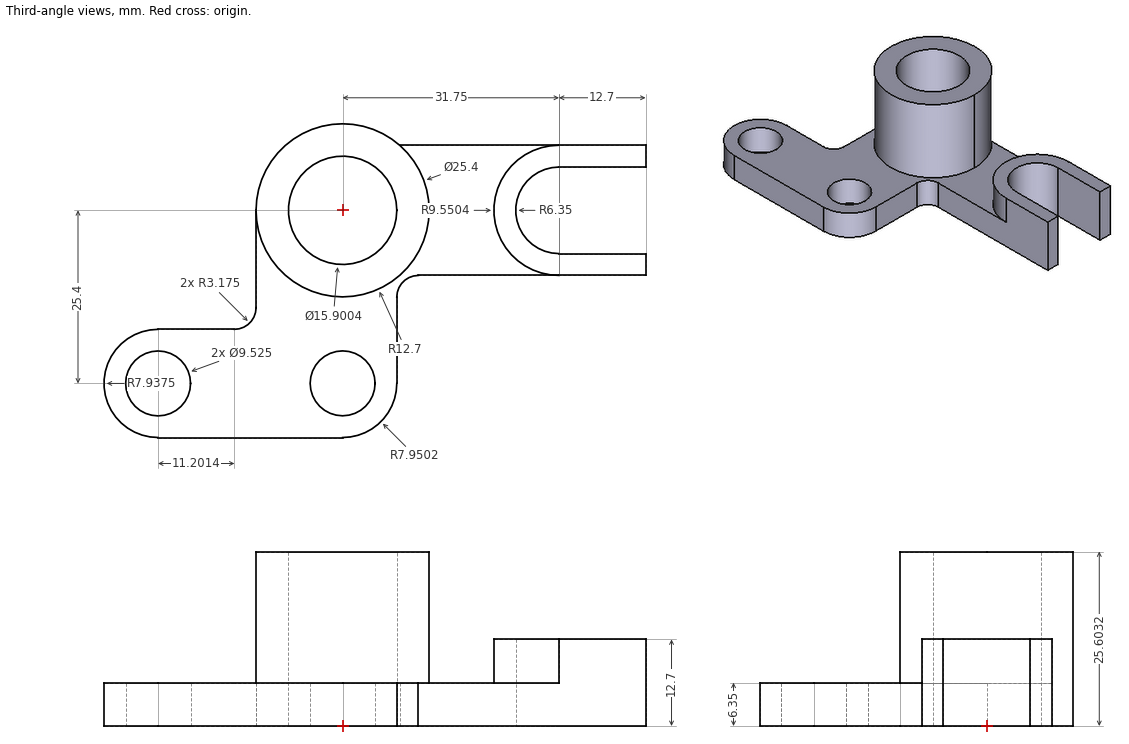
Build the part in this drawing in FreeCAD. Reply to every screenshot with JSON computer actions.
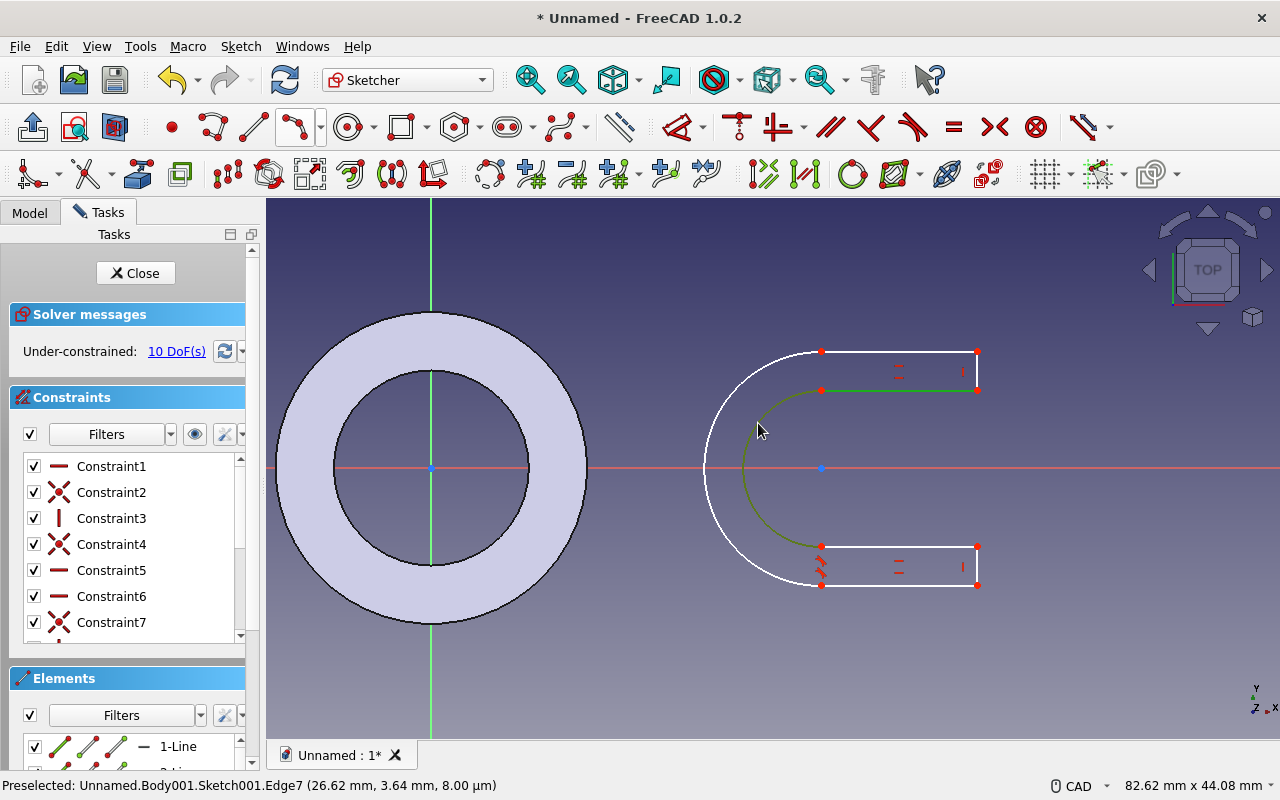
{"action": "left_click", "coordinate": [913, 128]}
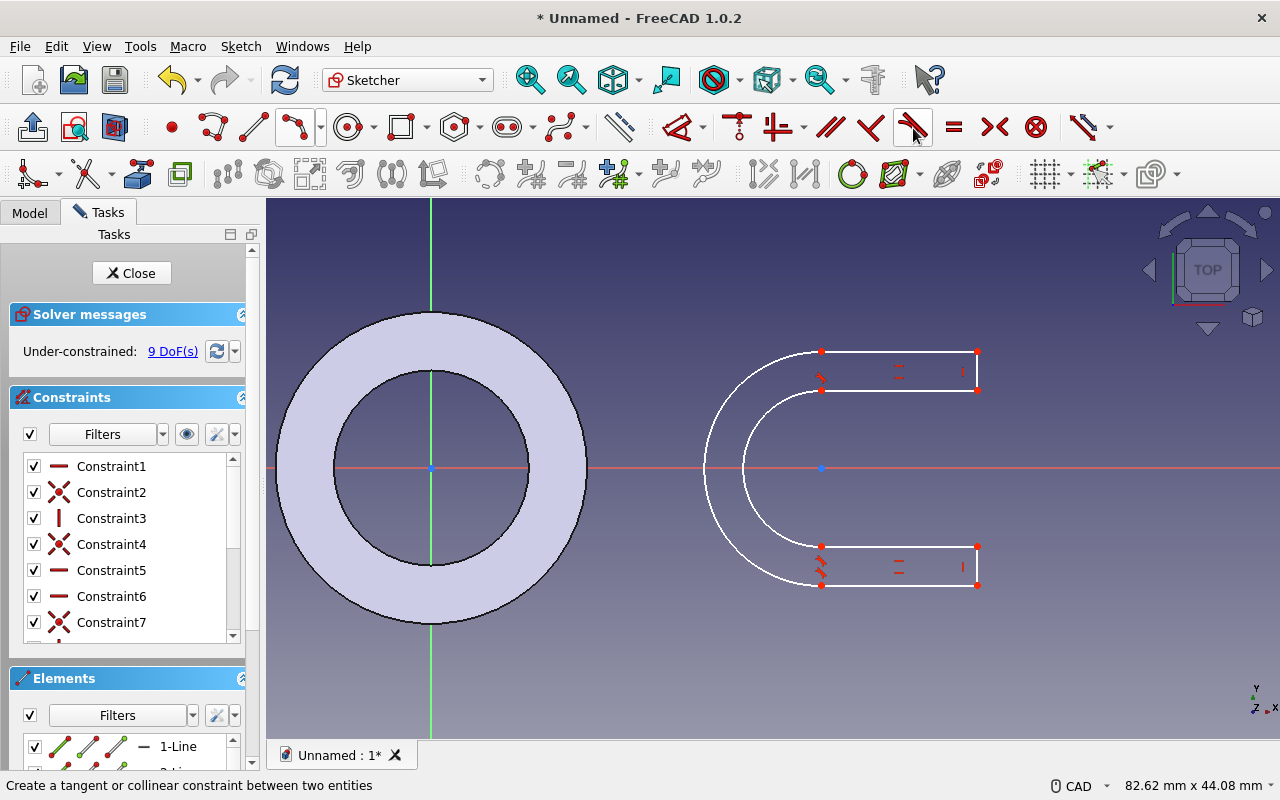
{"action": "left_click", "coordinate": [930, 352]}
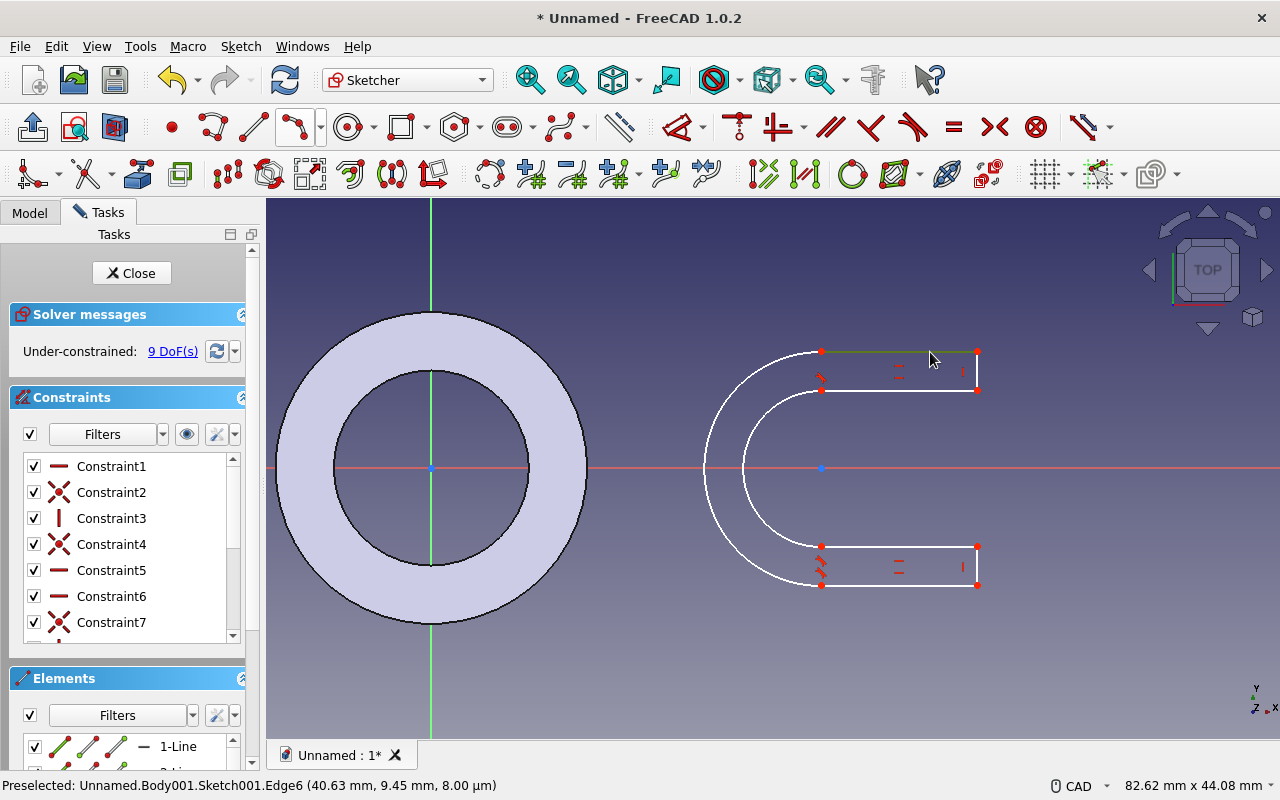
{"action": "left_click", "coordinate": [727, 400]}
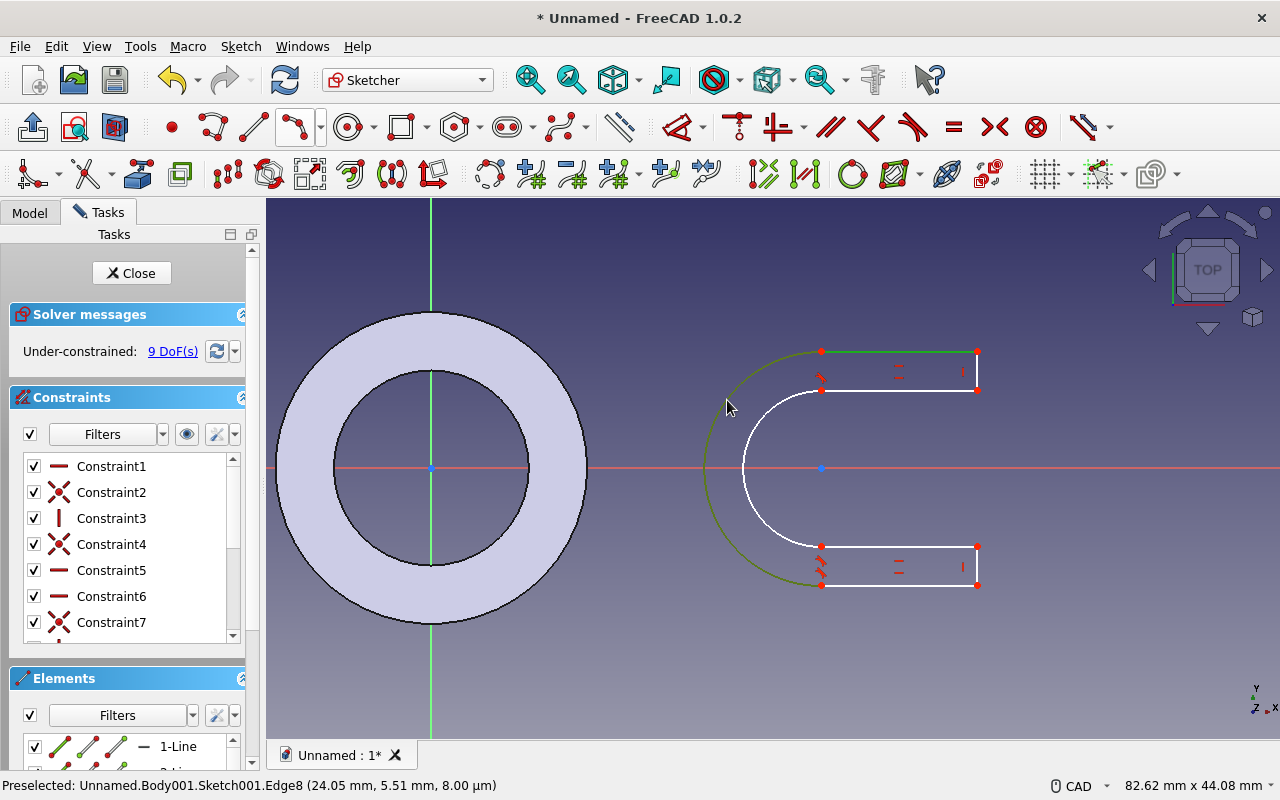
{"action": "key", "text": "t"}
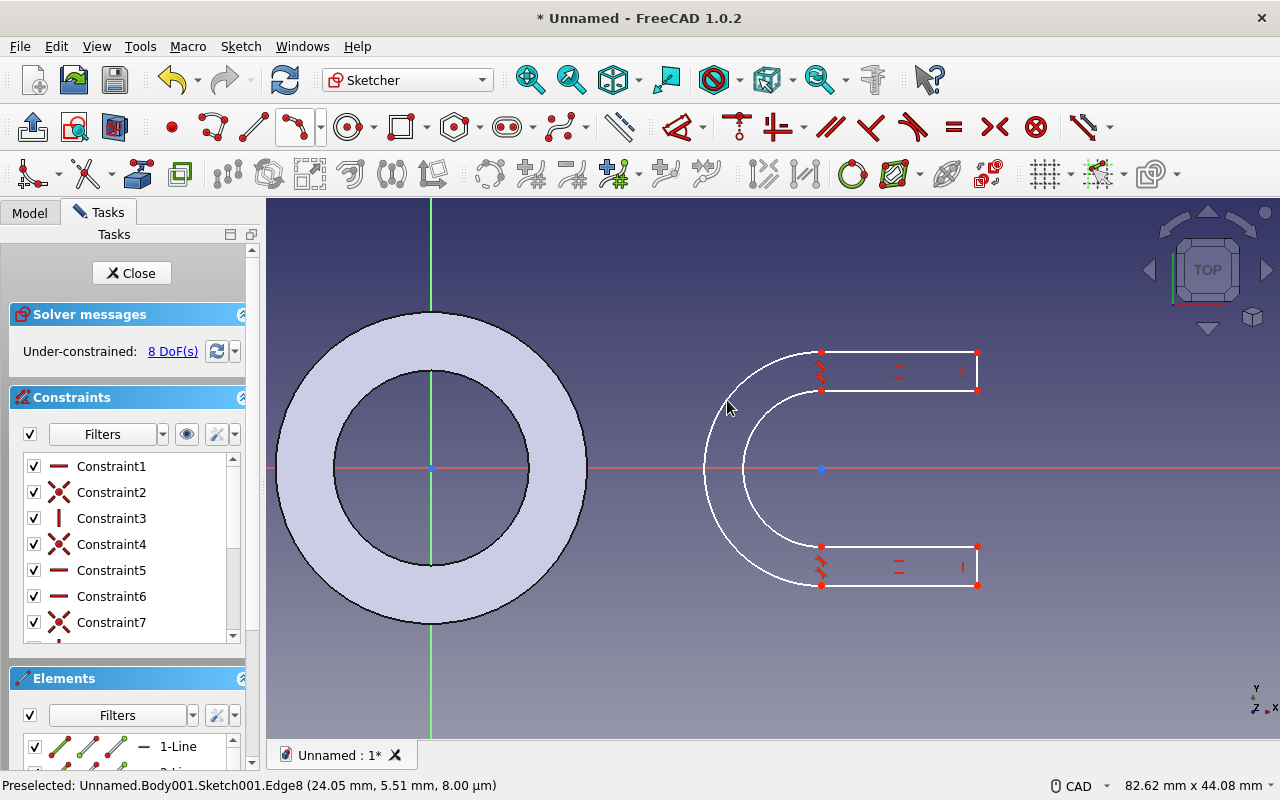
{"action": "left_click", "coordinate": [758, 423]}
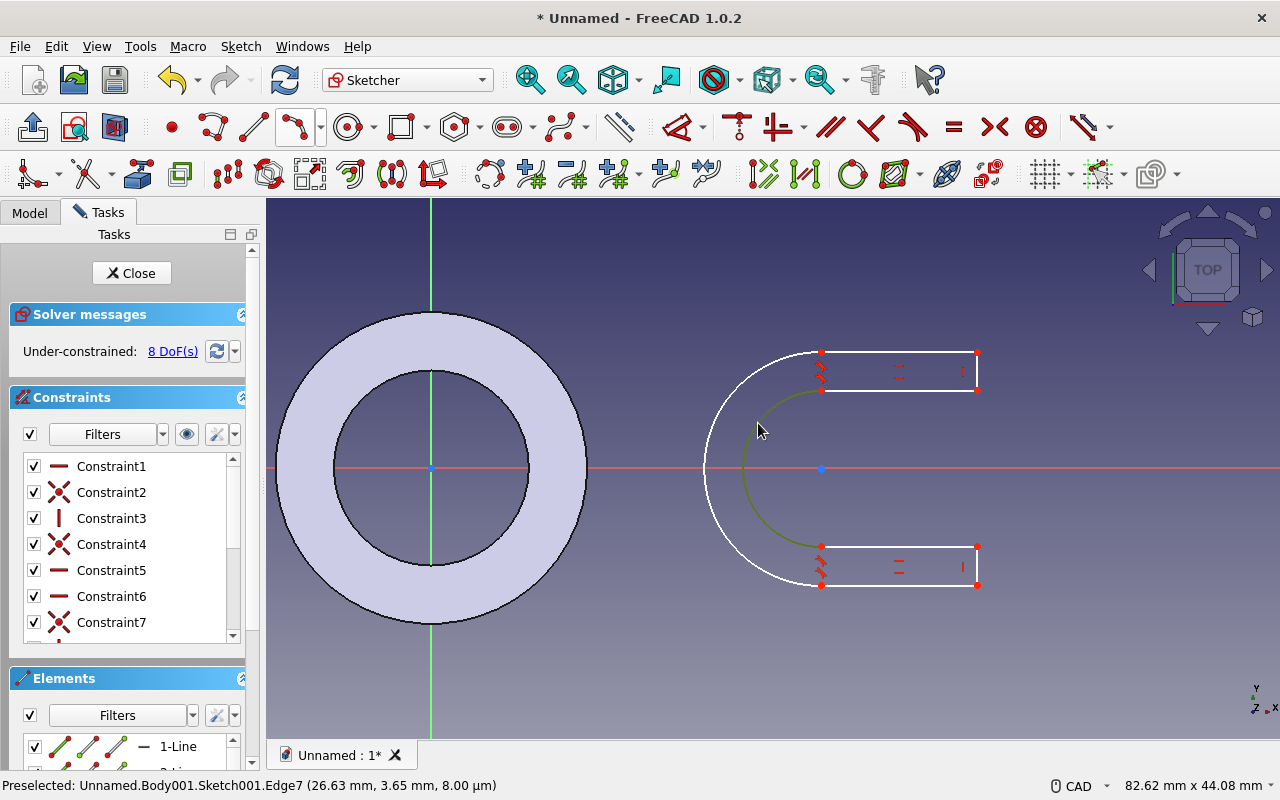
{"action": "left_click", "coordinate": [727, 400]}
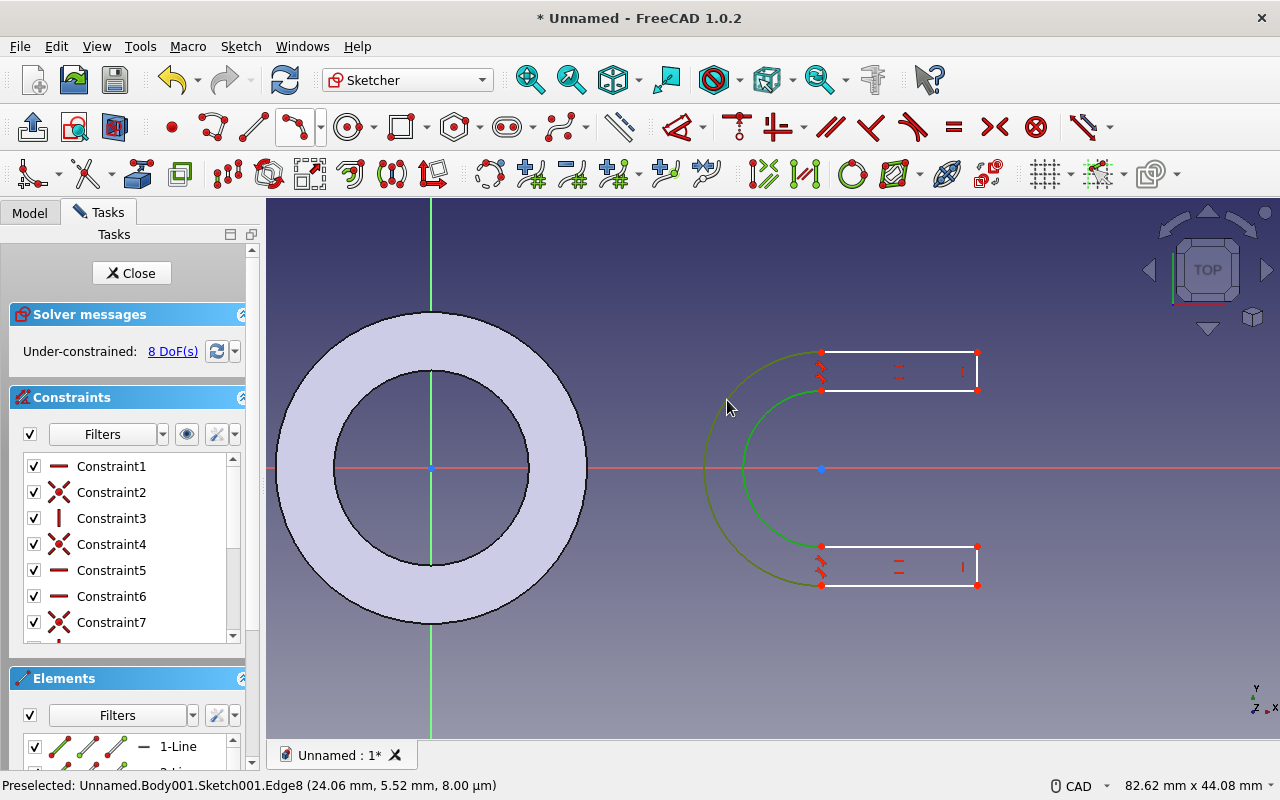
{"action": "key", "text": "c"}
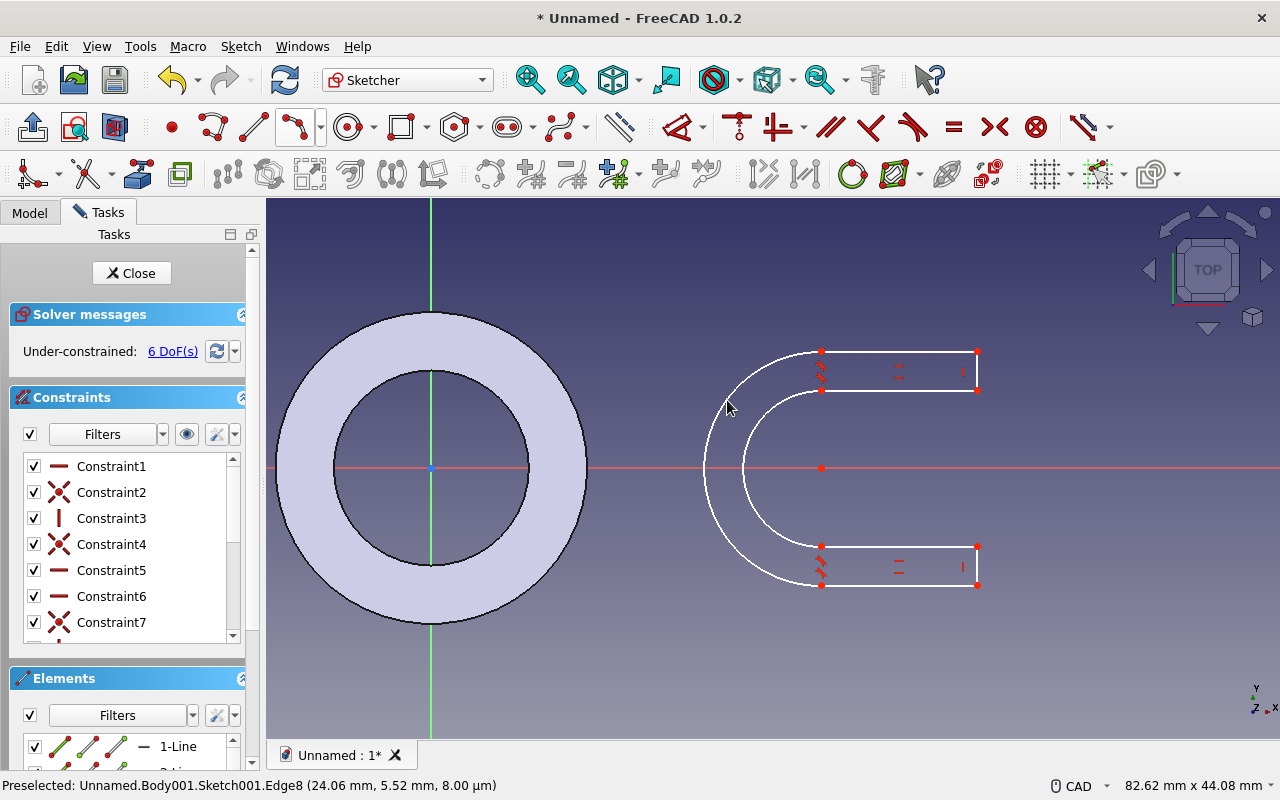
{"action": "left_click", "coordinate": [821, 469]}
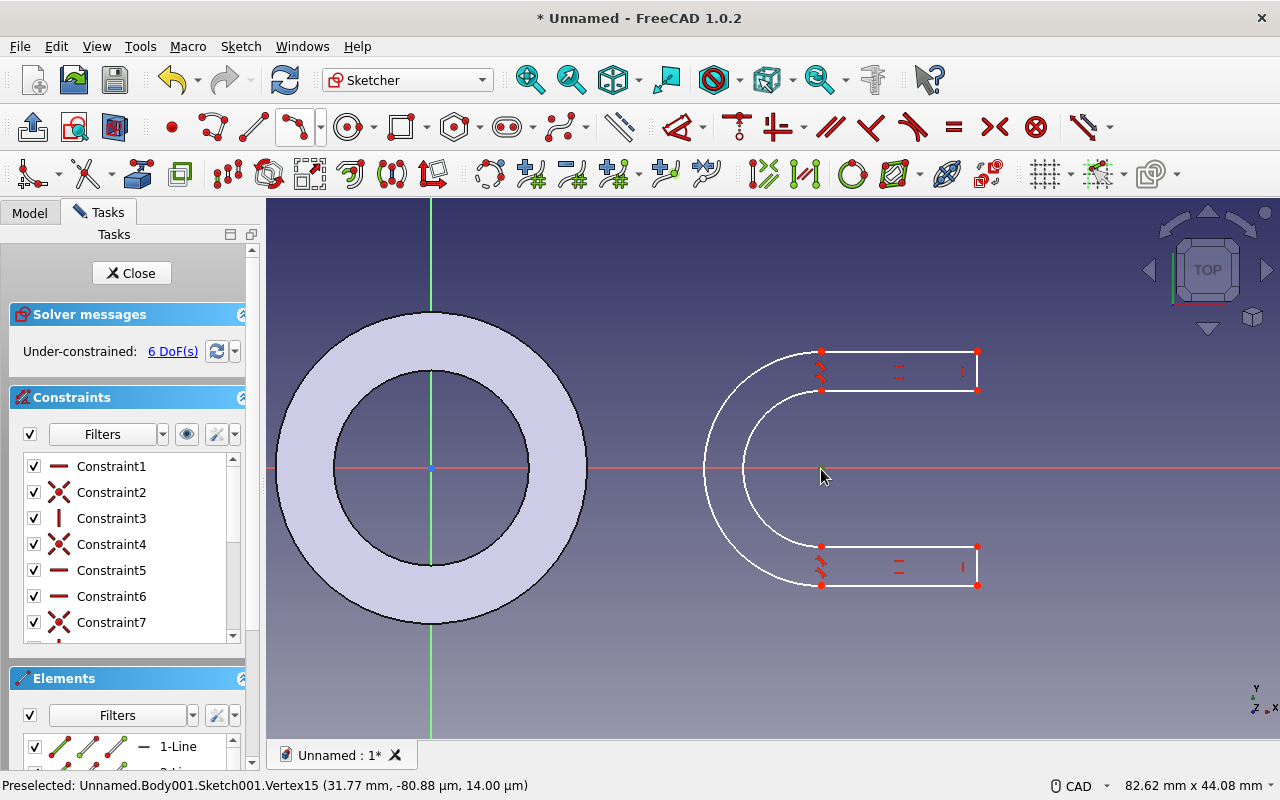
{"action": "left_click", "coordinate": [353, 468]}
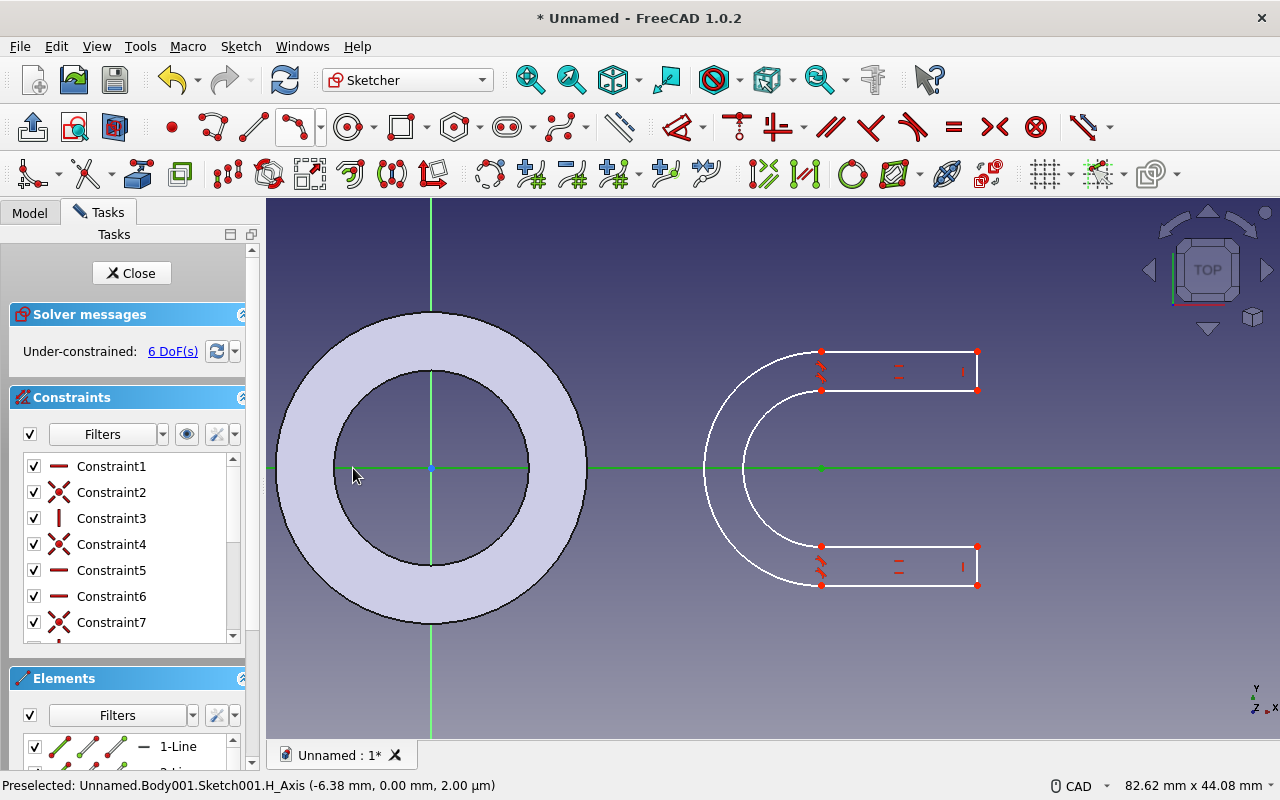
{"action": "left_click", "coordinate": [737, 128]}